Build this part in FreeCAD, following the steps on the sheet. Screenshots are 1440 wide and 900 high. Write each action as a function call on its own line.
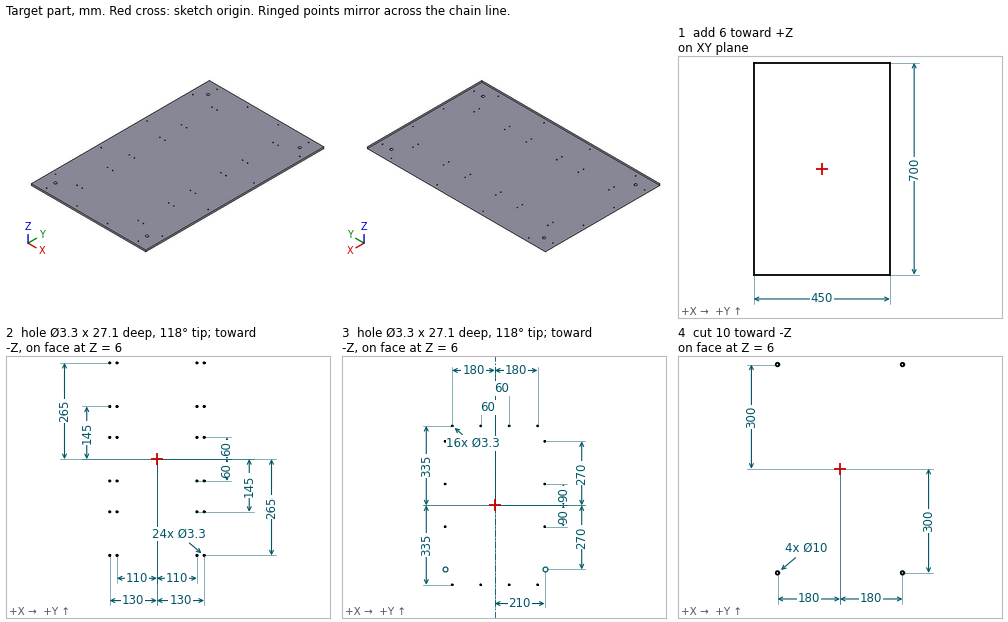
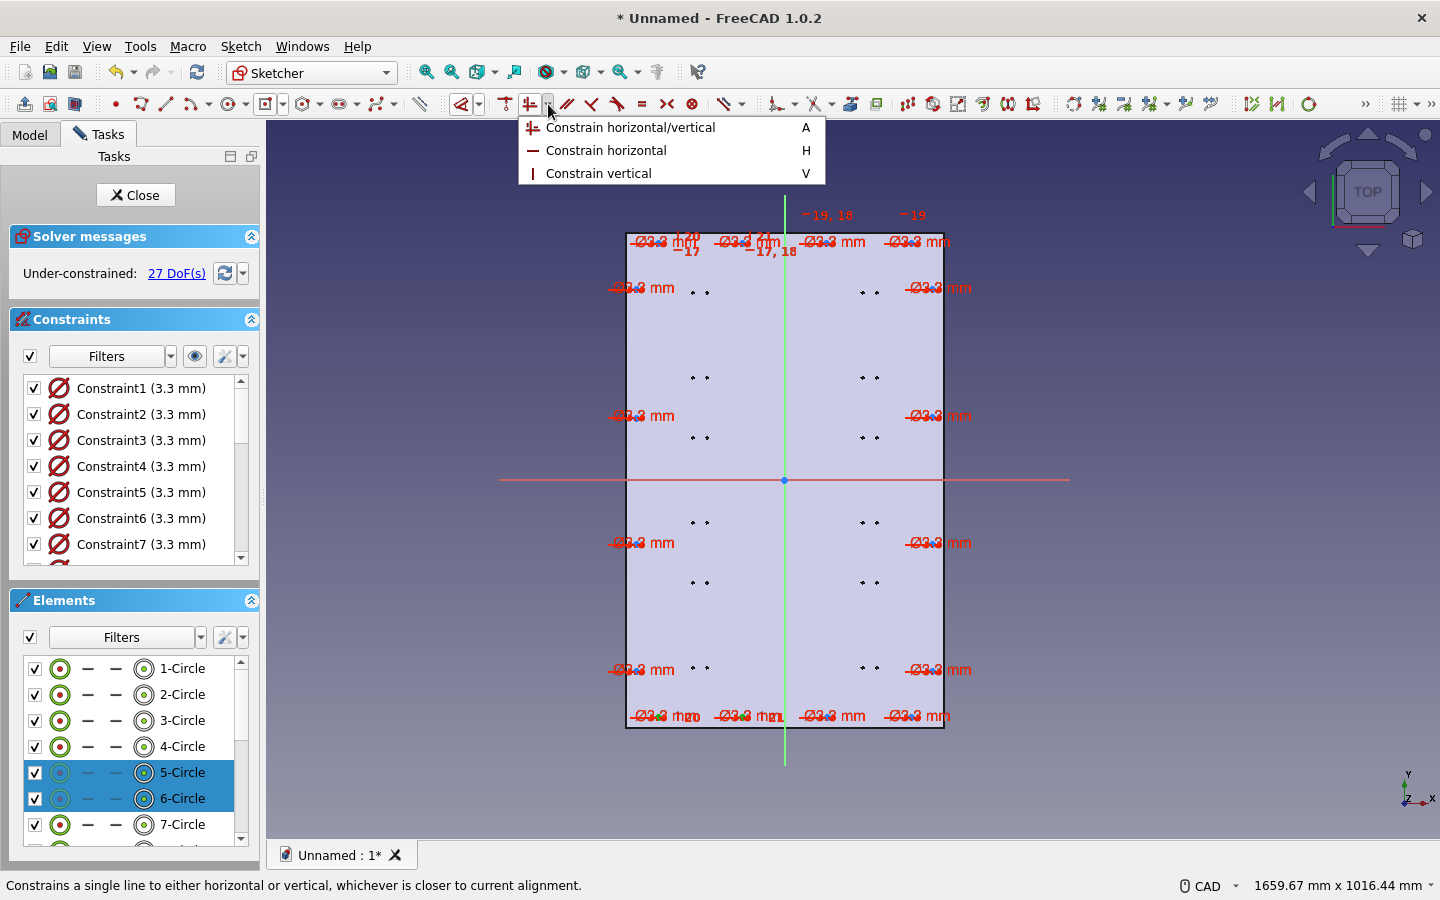
click(672, 150)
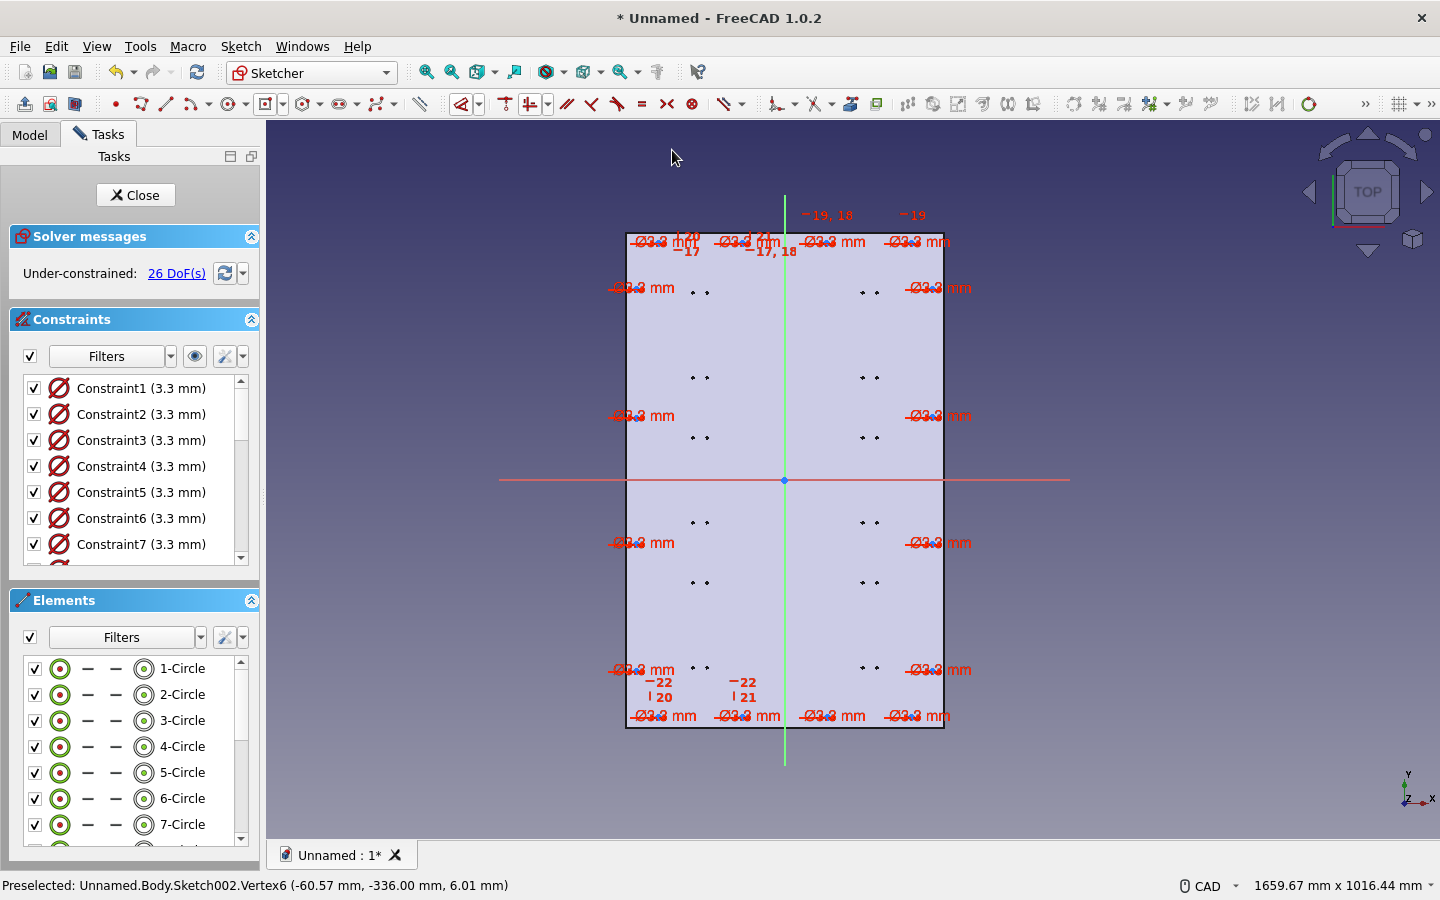
click(827, 244)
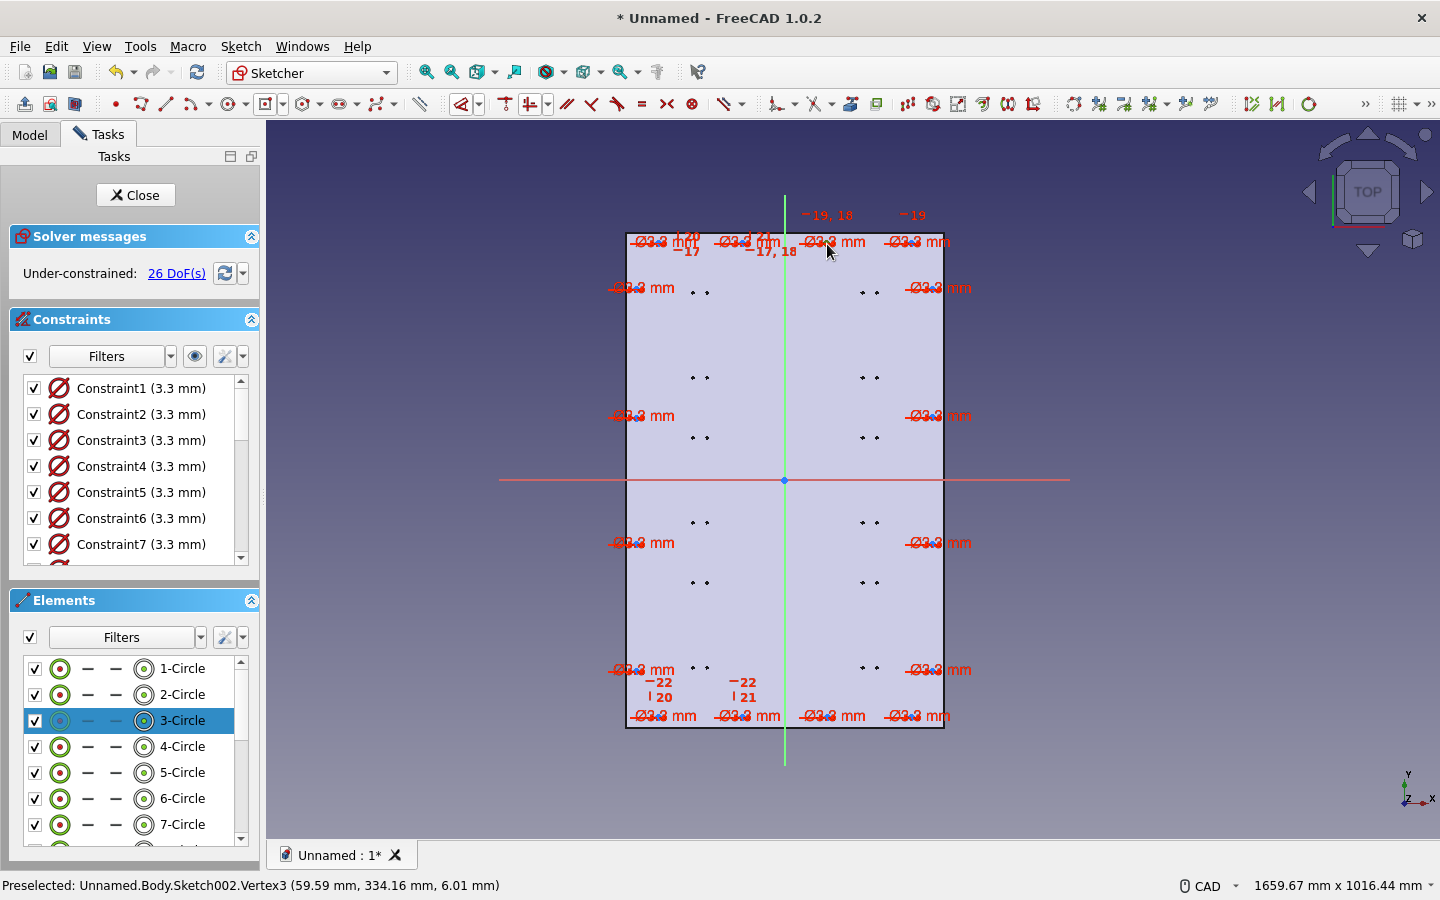
click(827, 718)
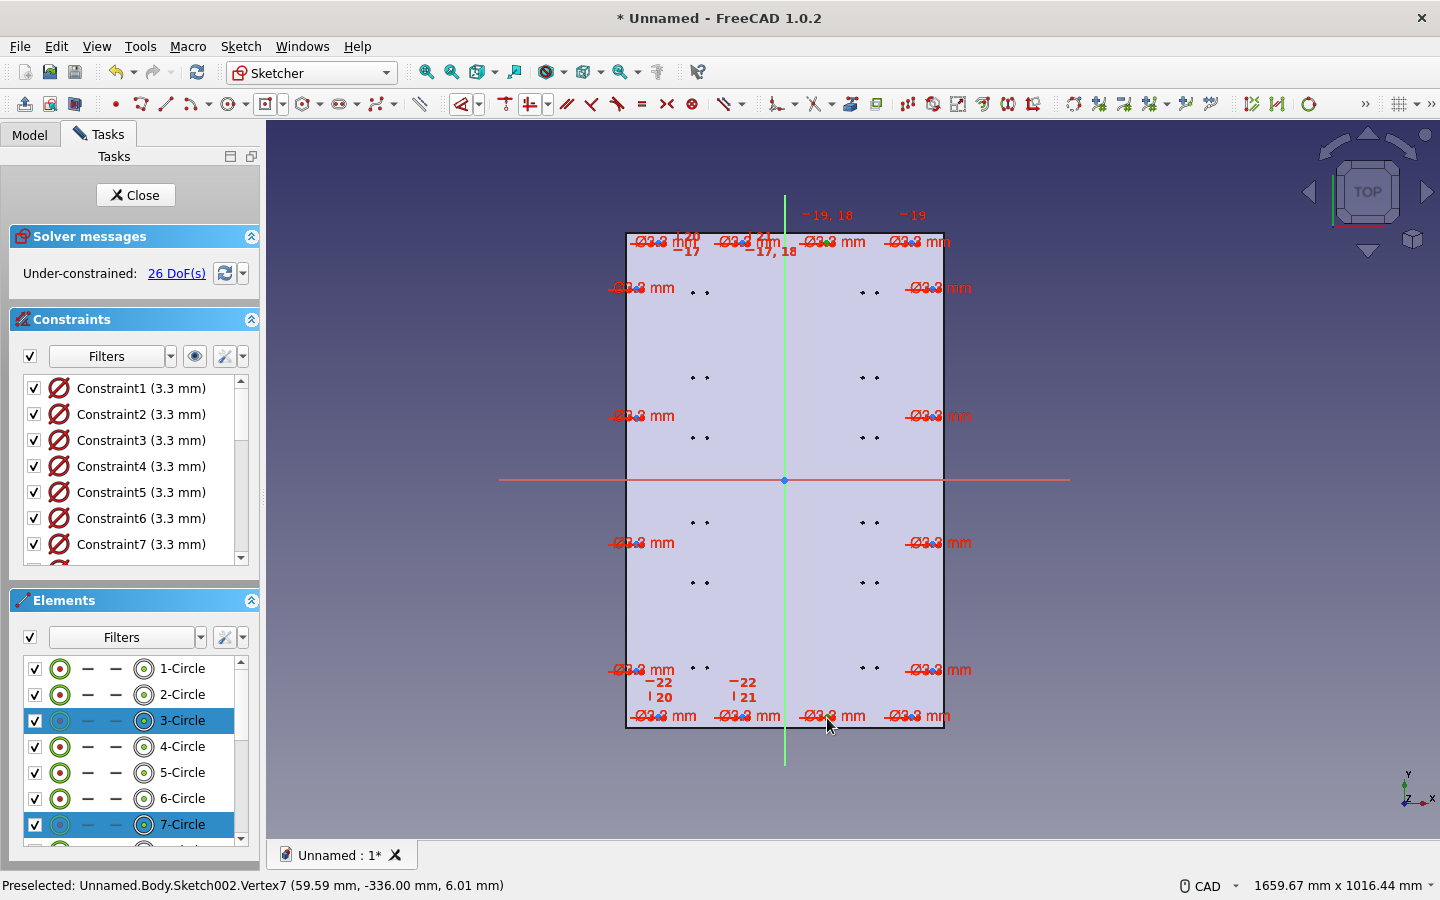
click(548, 104)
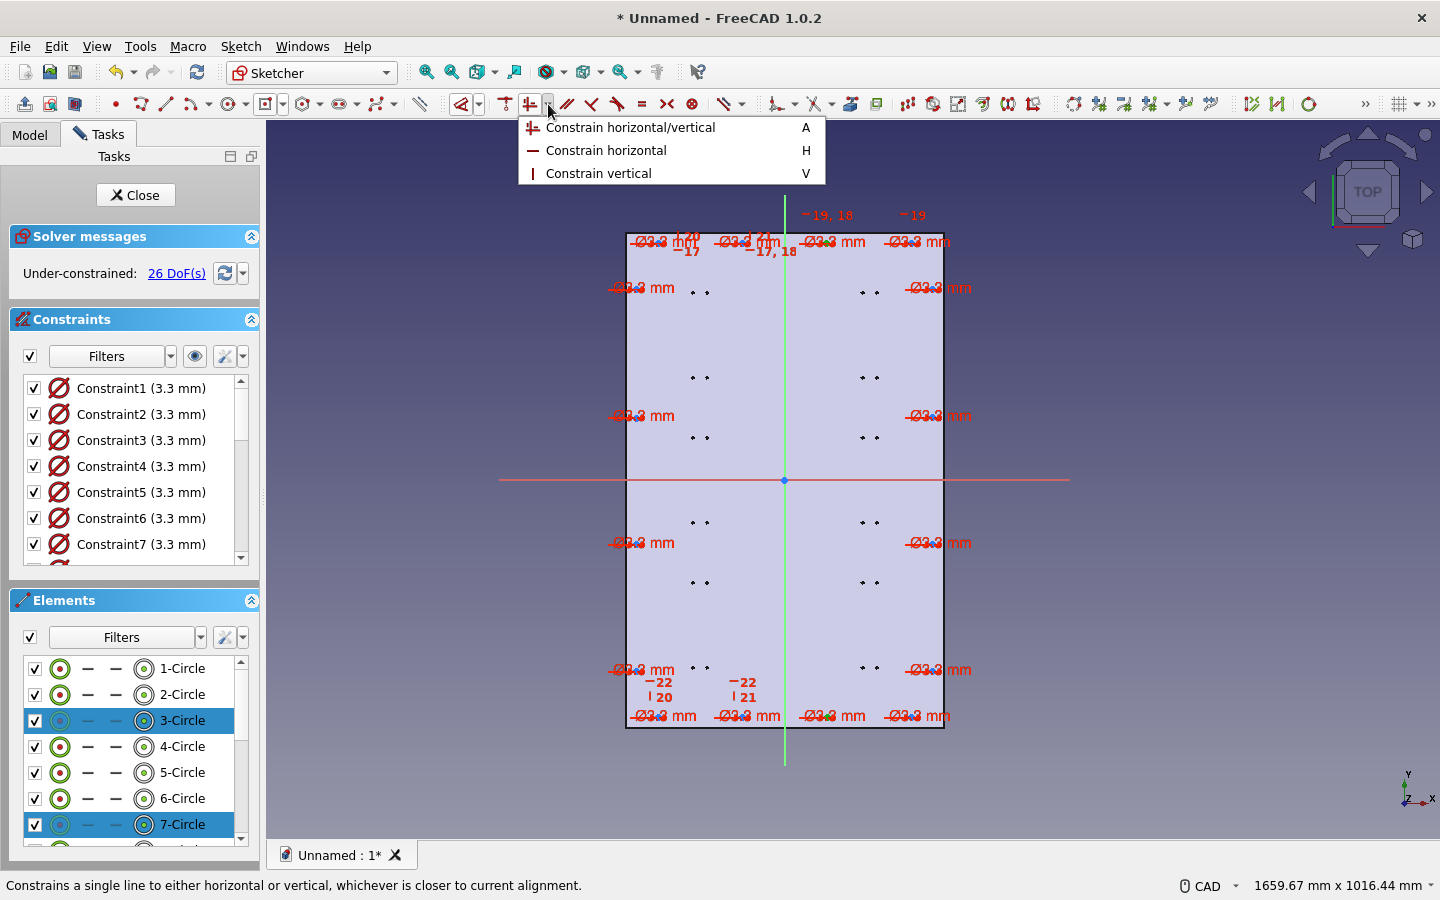
click(672, 174)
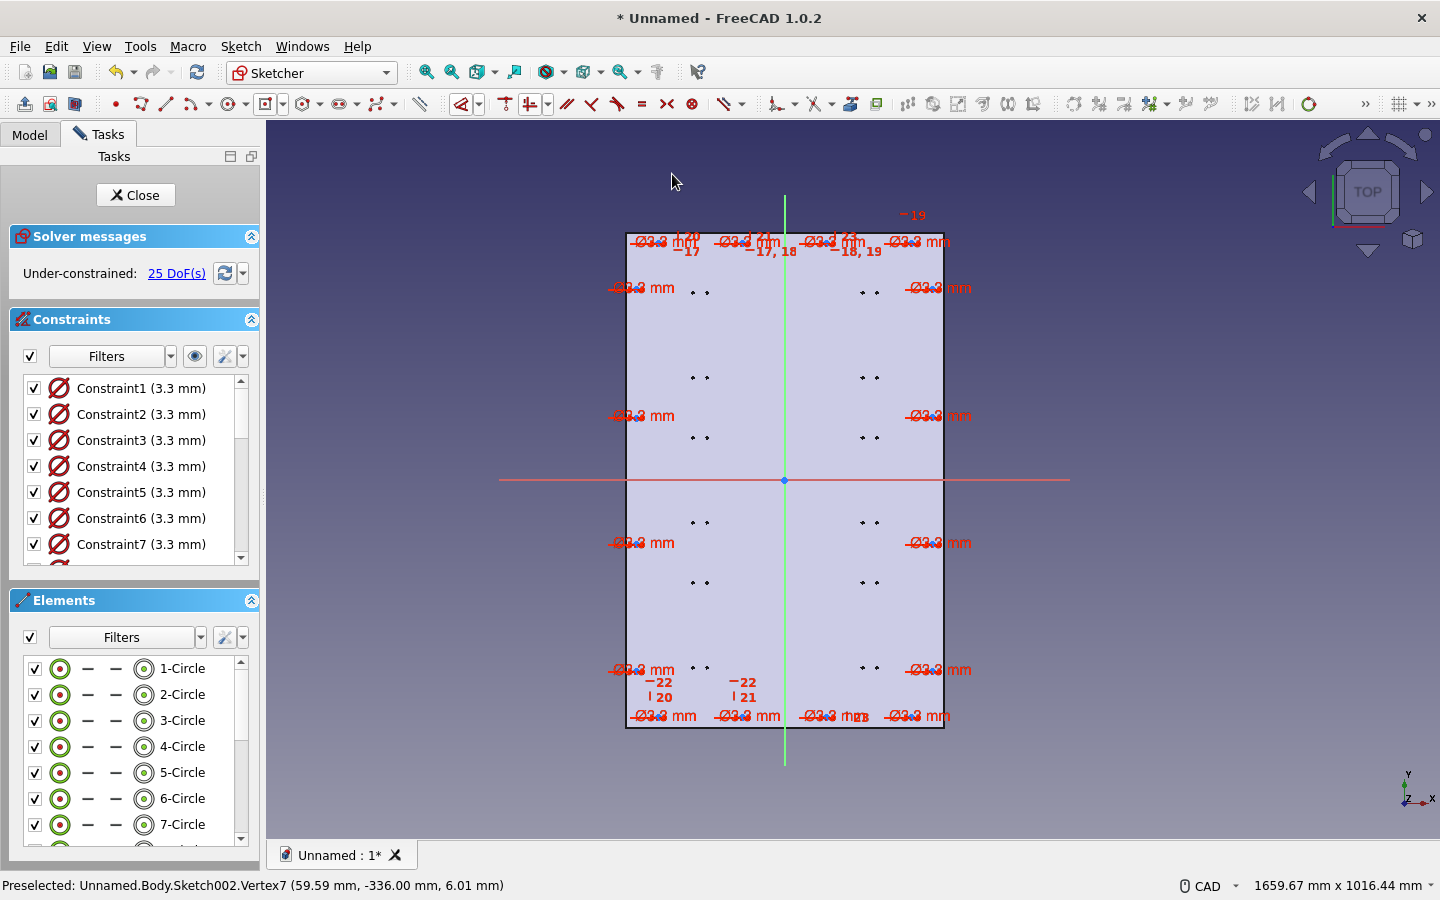
click(742, 718)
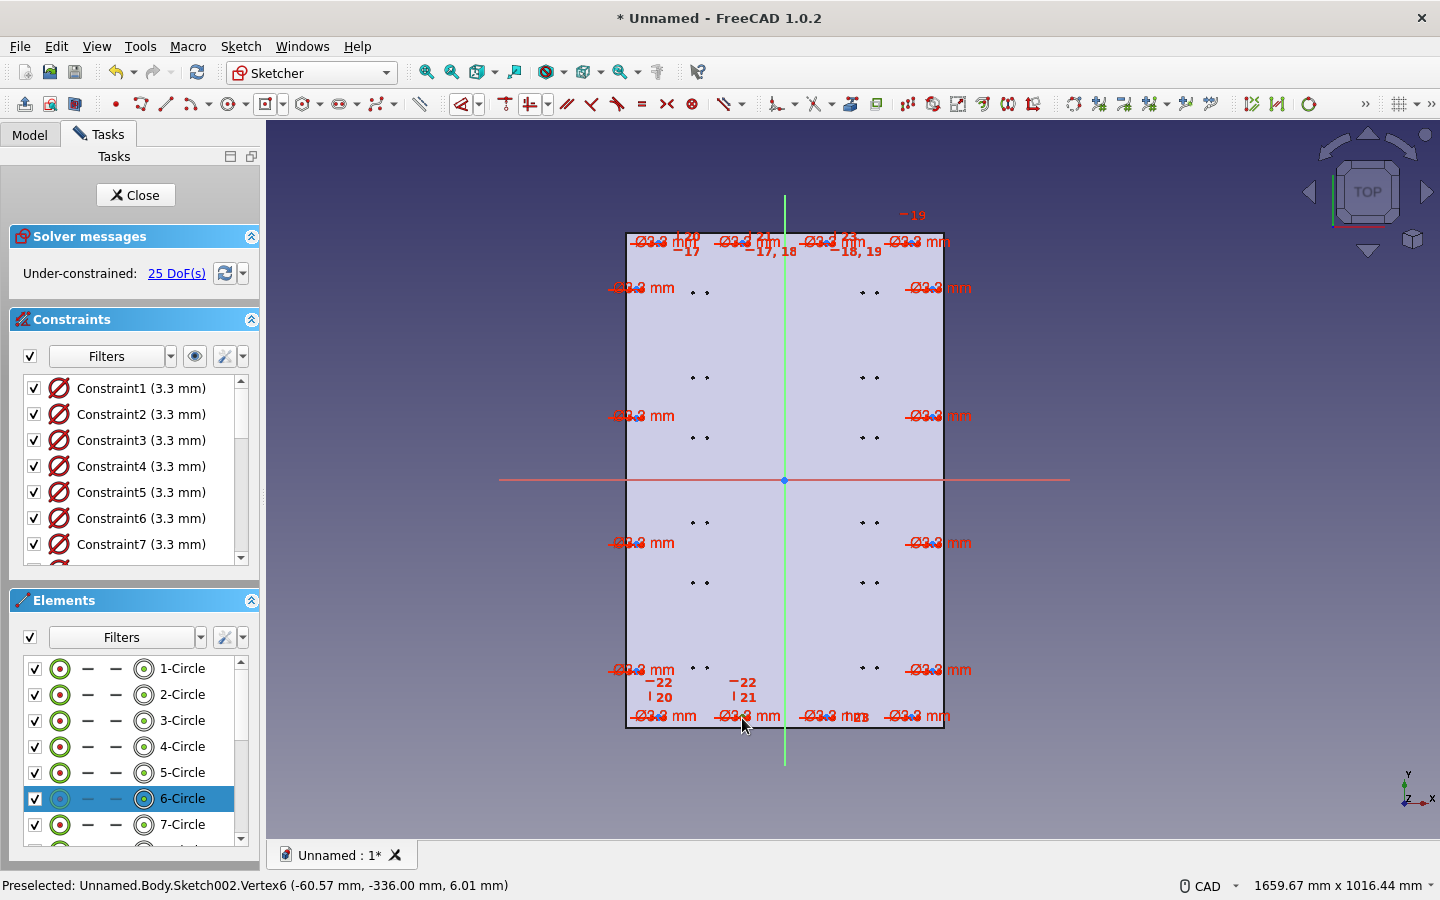
click(827, 718)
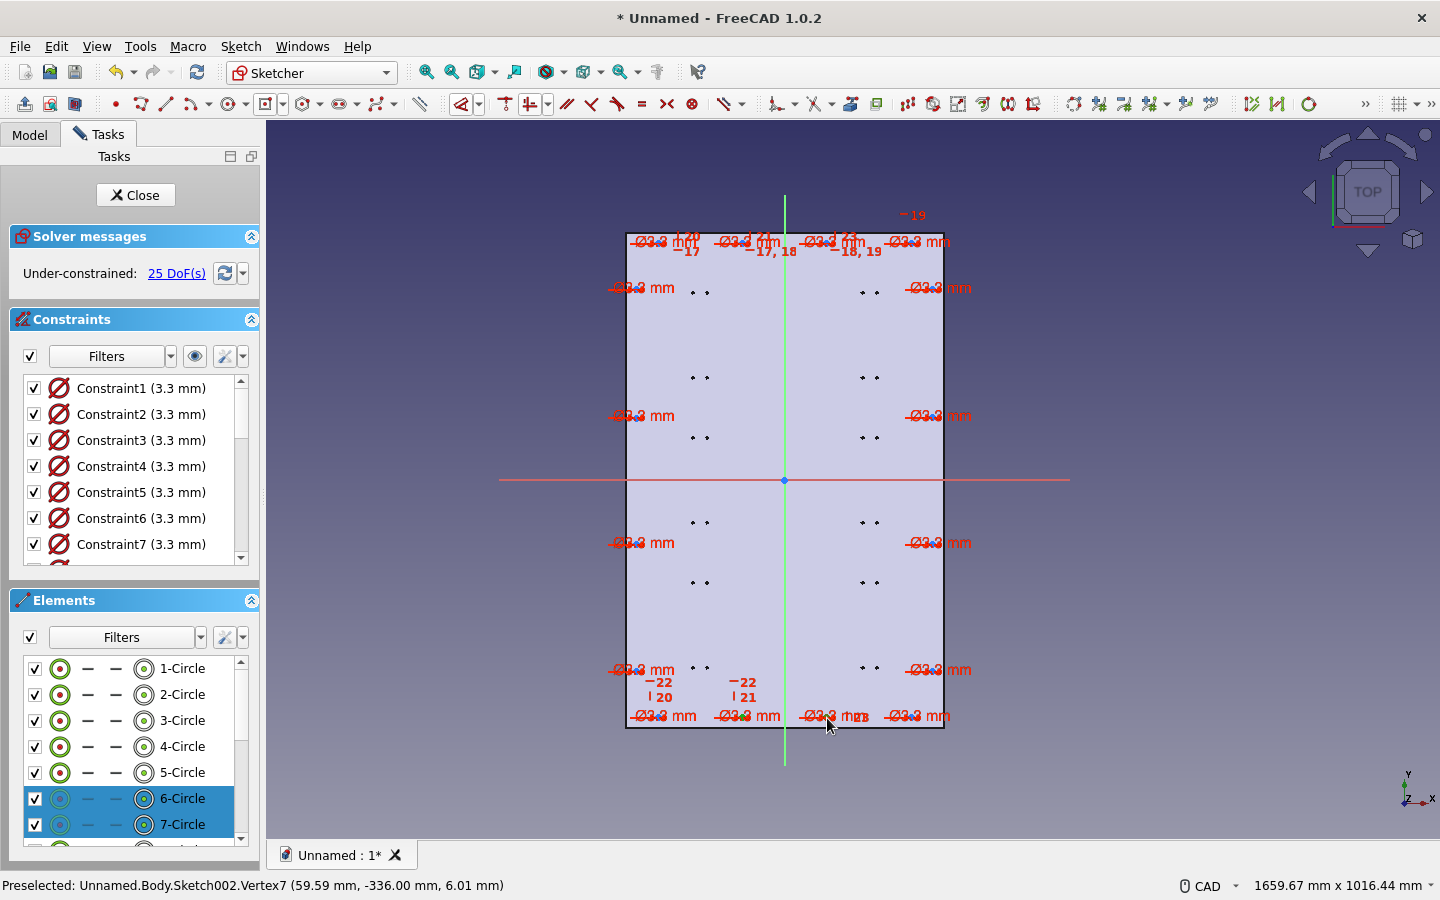
click(548, 104)